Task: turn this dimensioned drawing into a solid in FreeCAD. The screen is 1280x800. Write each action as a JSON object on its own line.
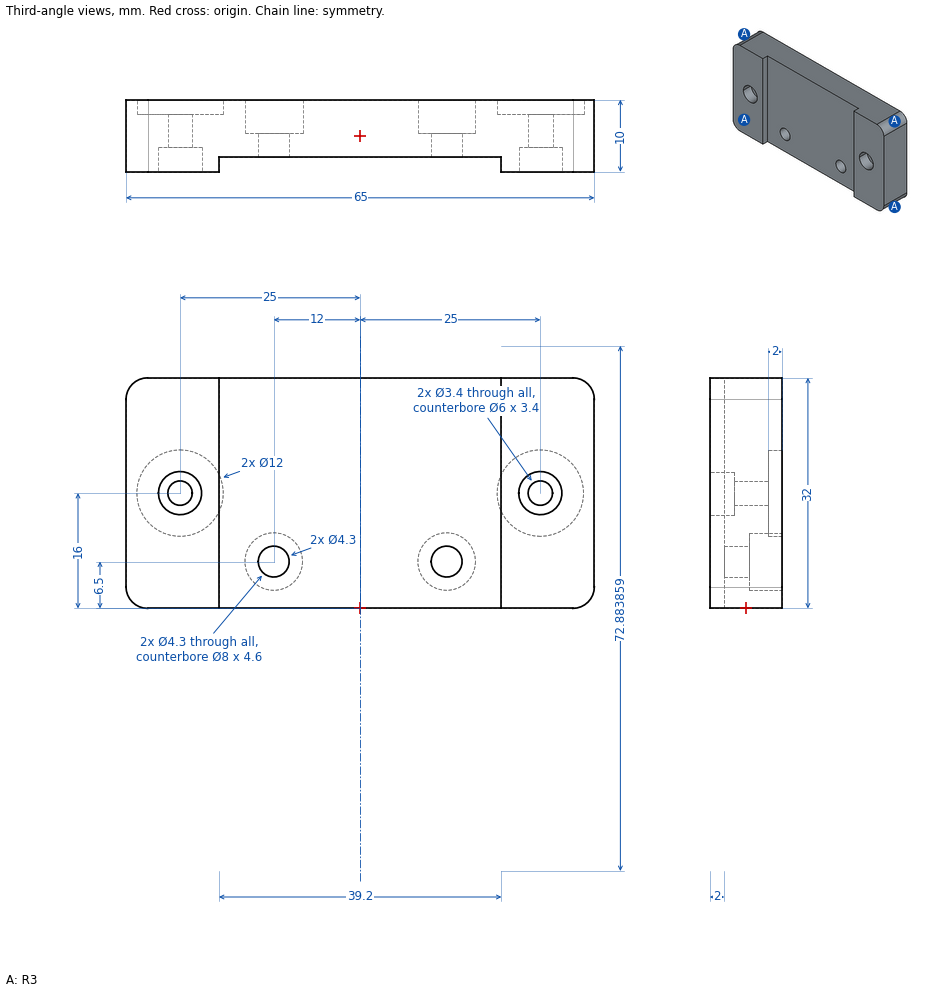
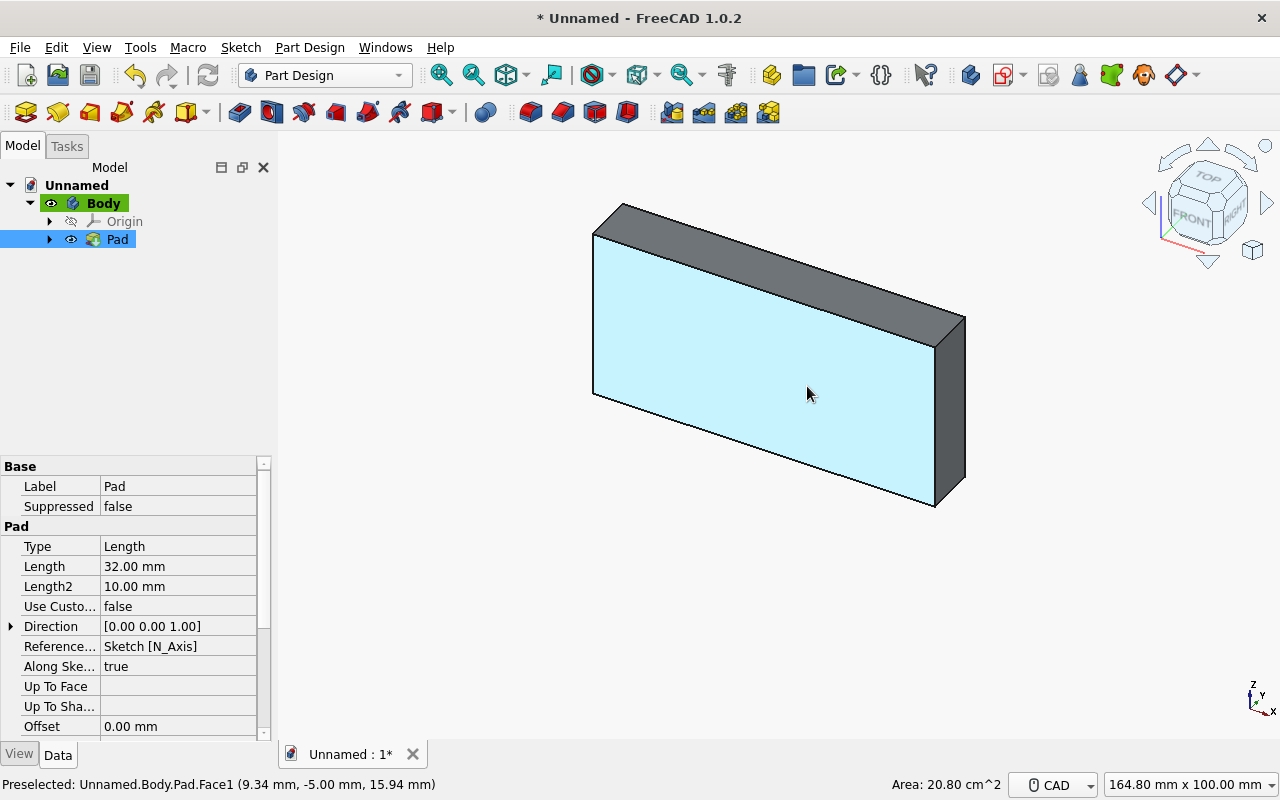
{"action": "left_click", "coordinate": [1004, 76]}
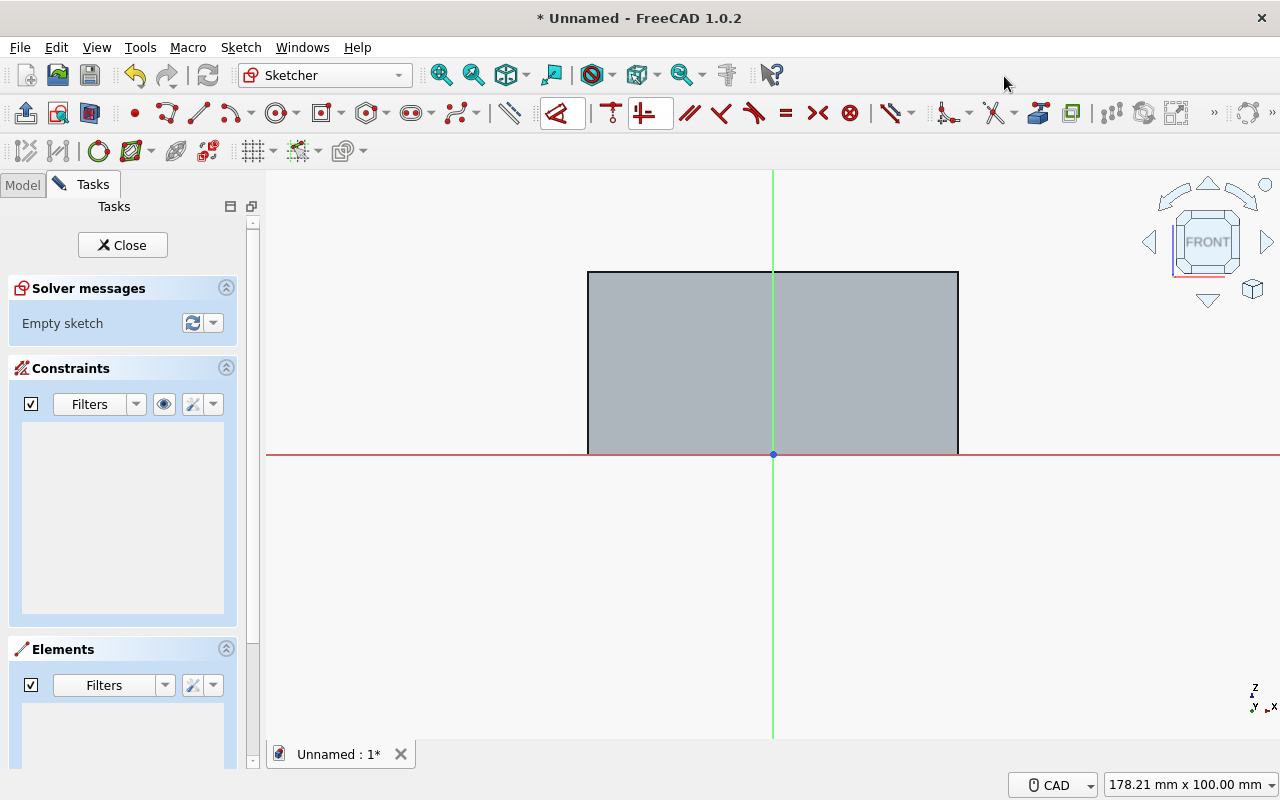
{"action": "scroll", "coordinate": [803, 419], "scroll_direction": "up", "scroll_amount": 6}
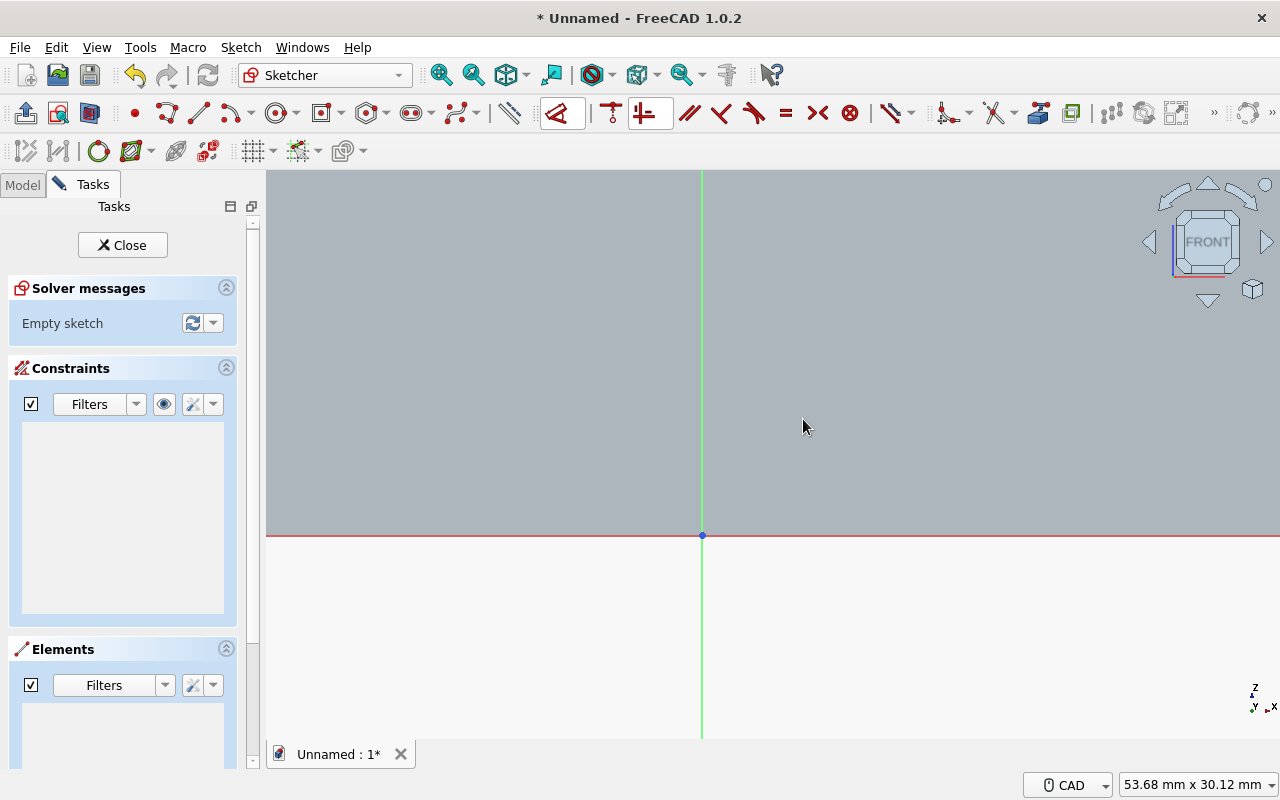
{"action": "left_click", "coordinate": [276, 114]}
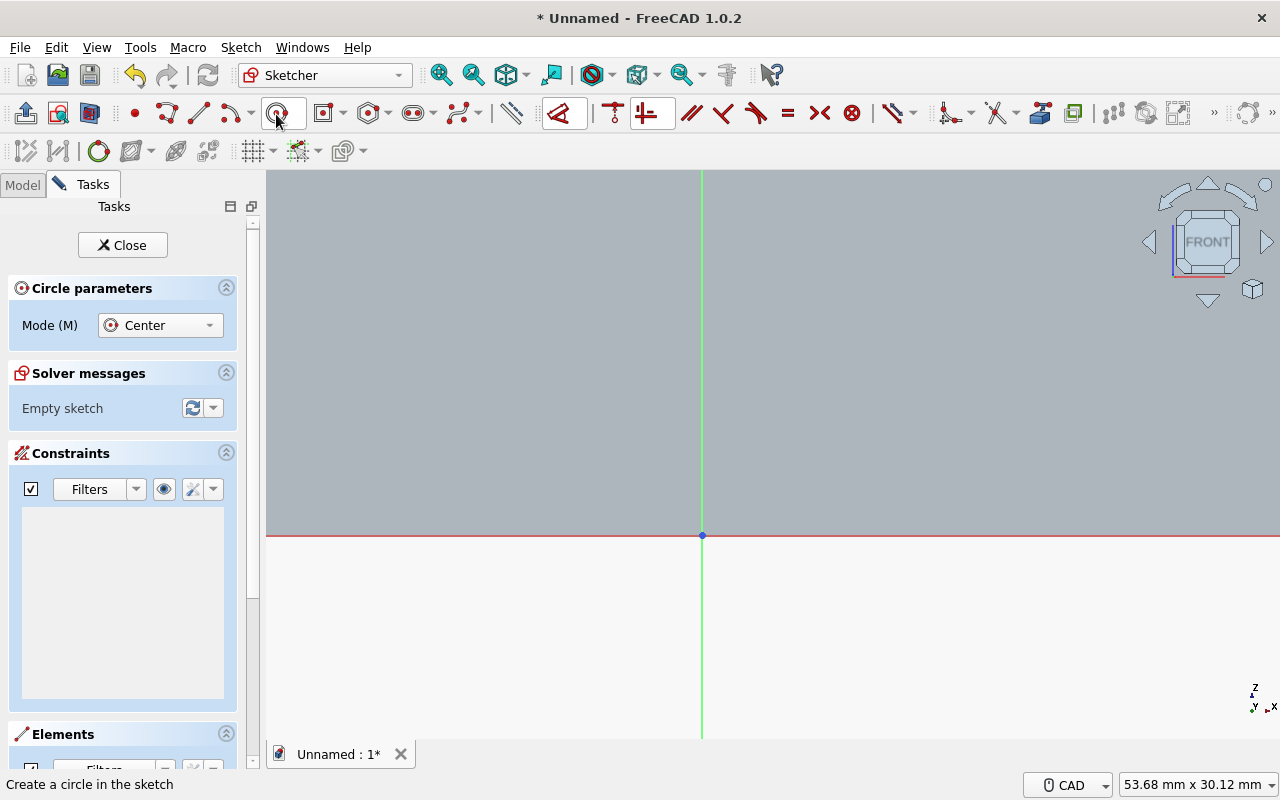
{"action": "left_click", "coordinate": [475, 413]}
{"action": "left_click", "coordinate": [504, 384]}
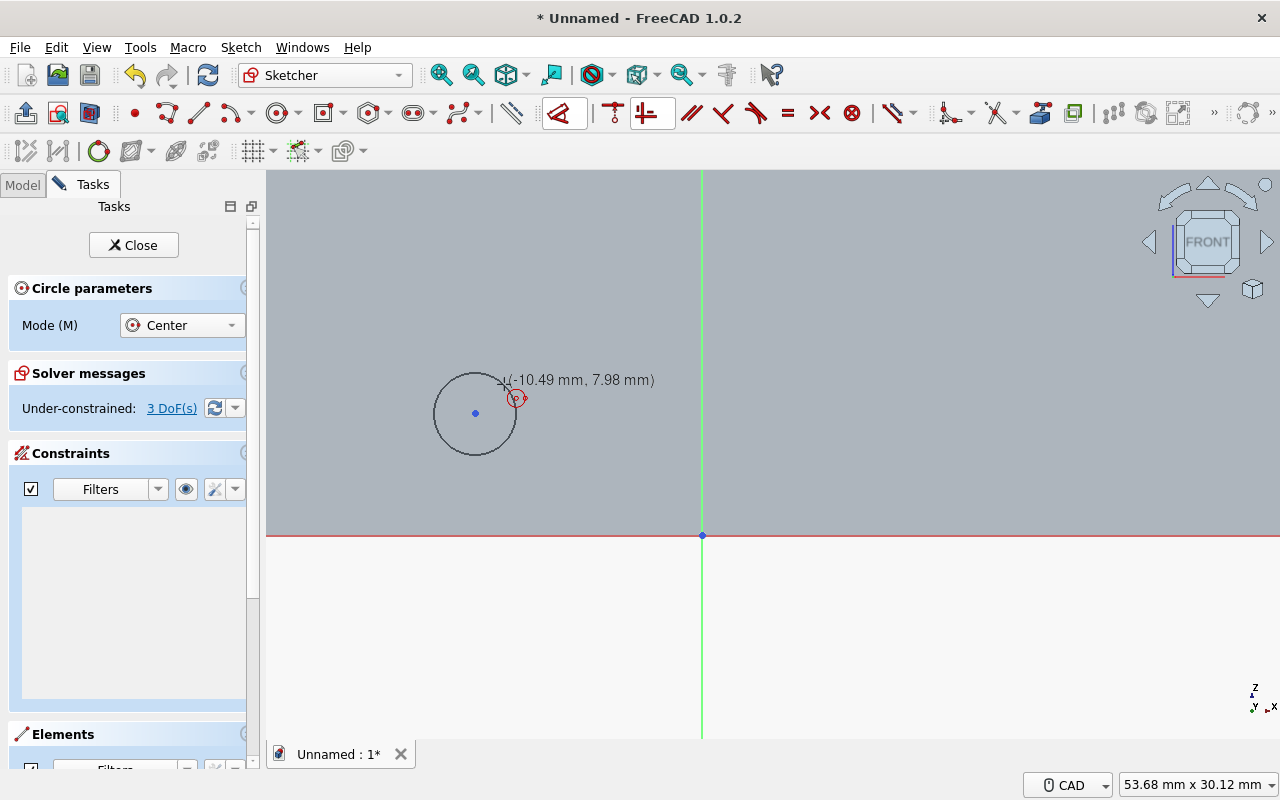
{"action": "left_click", "coordinate": [929, 413]}
{"action": "left_click", "coordinate": [958, 384]}
{"action": "key", "text": "Escape"}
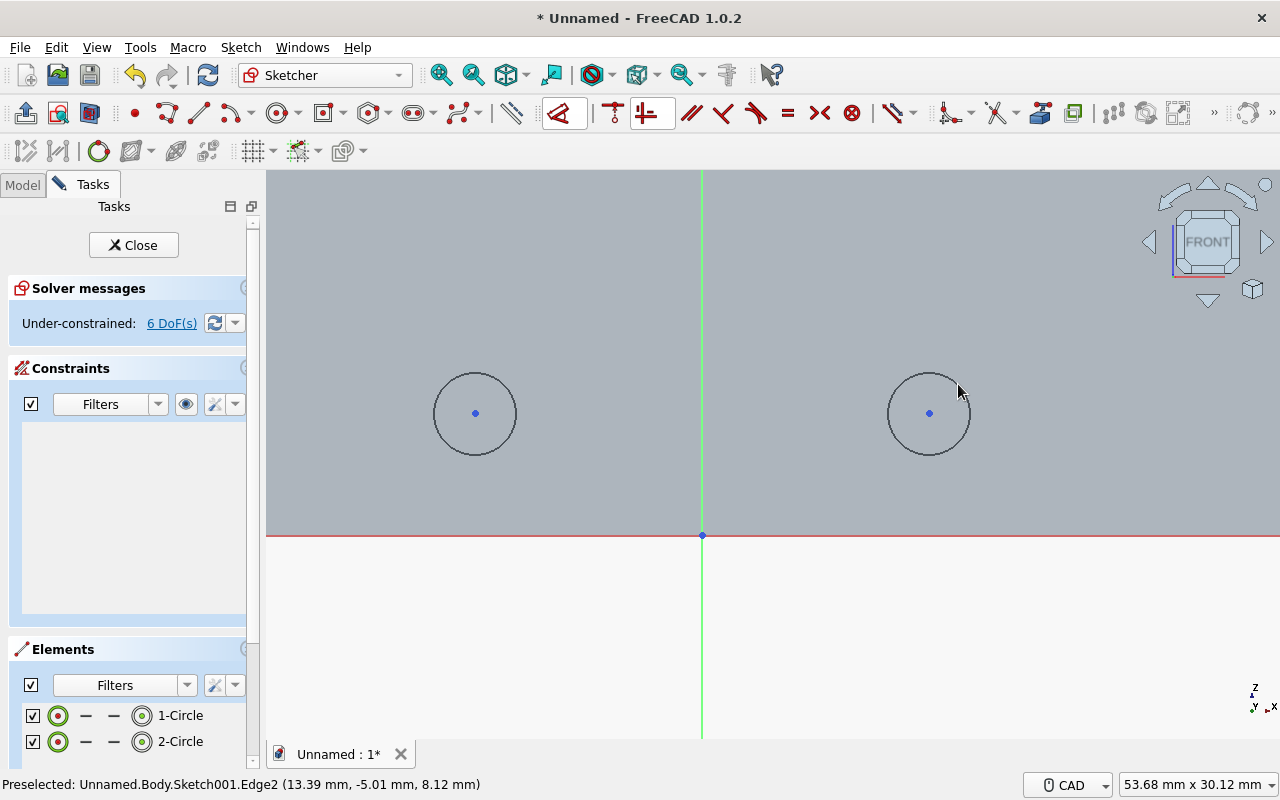
{"action": "left_click", "coordinate": [504, 385]}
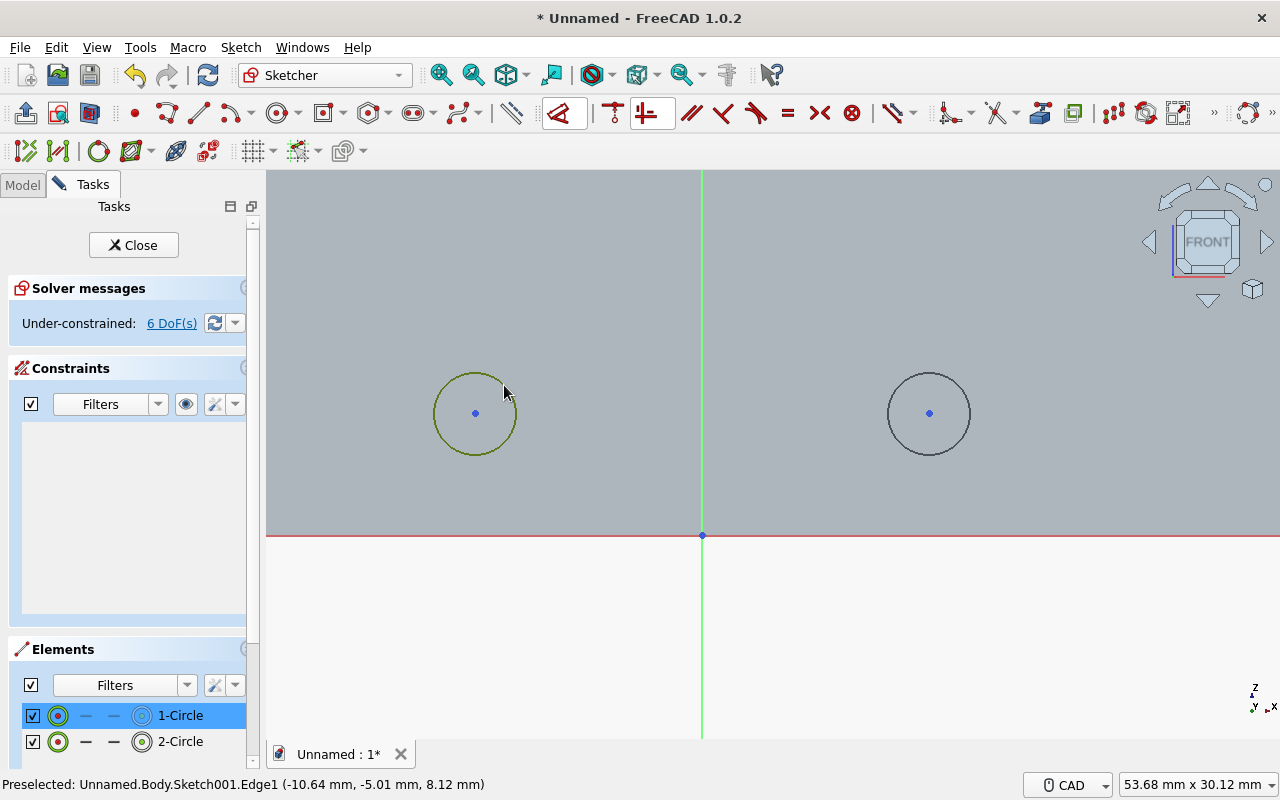
{"action": "left_click", "coordinate": [958, 385]}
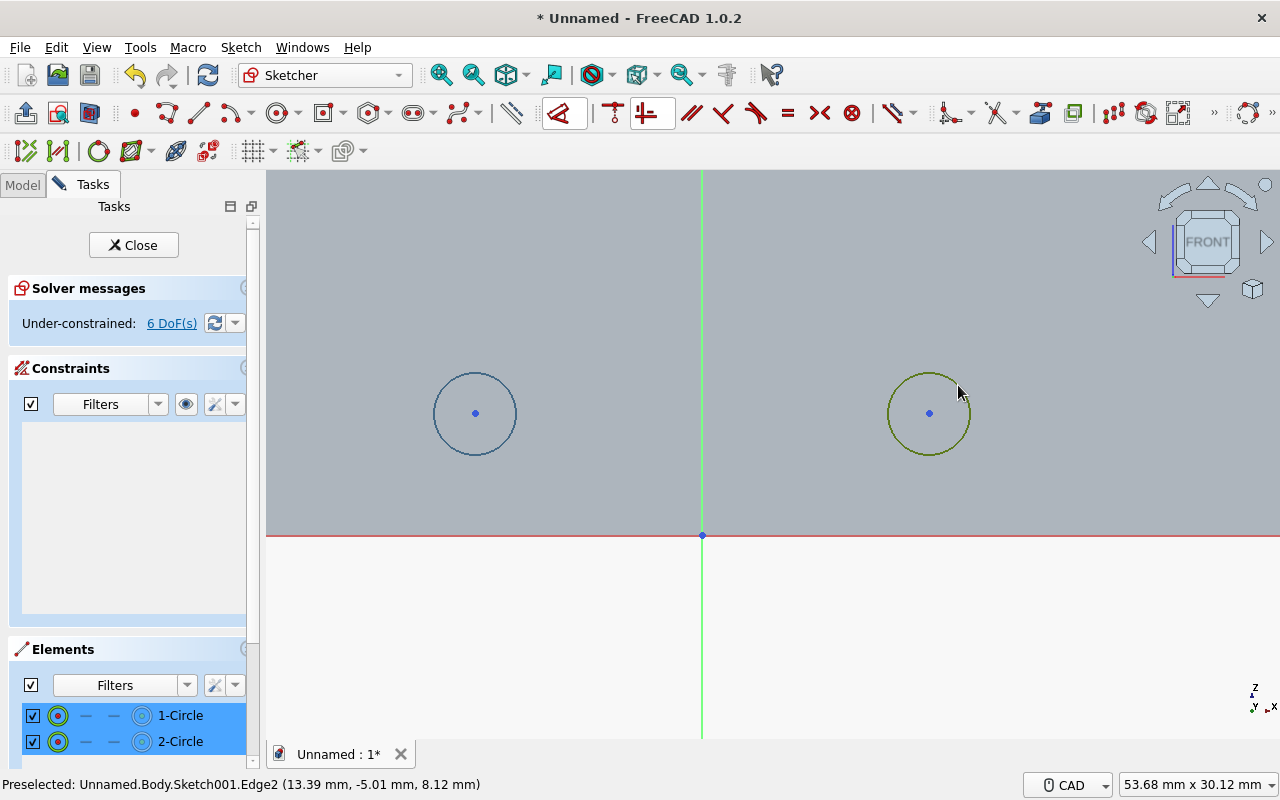
{"action": "left_click", "coordinate": [788, 114]}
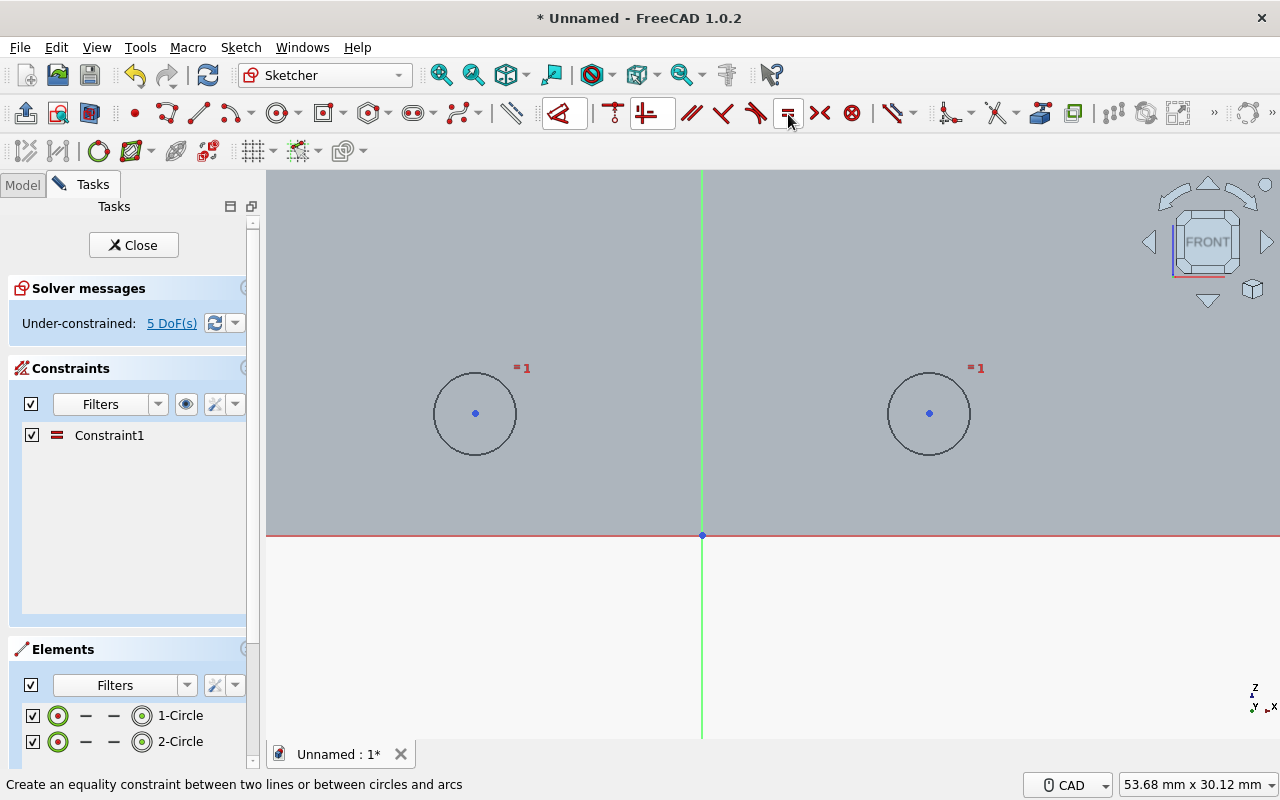
{"action": "left_click", "coordinate": [475, 414]}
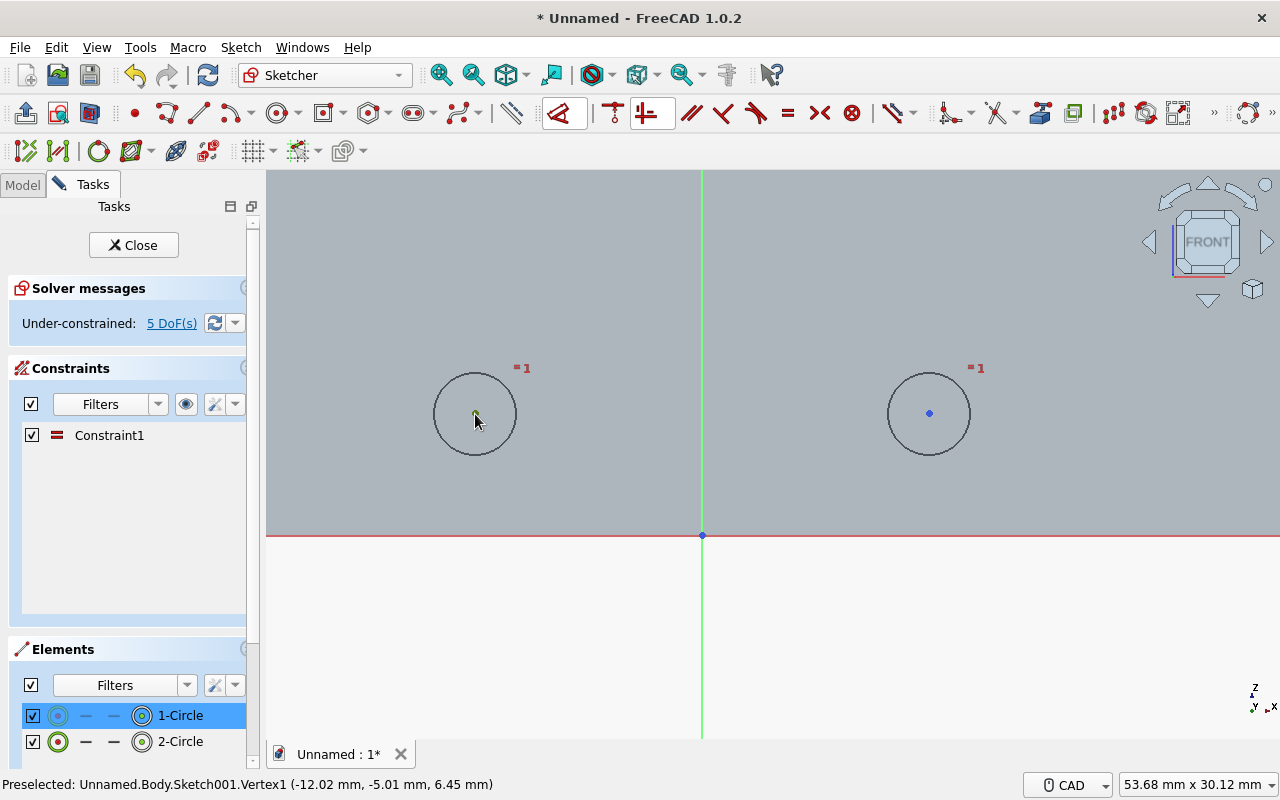
{"action": "left_click", "coordinate": [929, 414]}